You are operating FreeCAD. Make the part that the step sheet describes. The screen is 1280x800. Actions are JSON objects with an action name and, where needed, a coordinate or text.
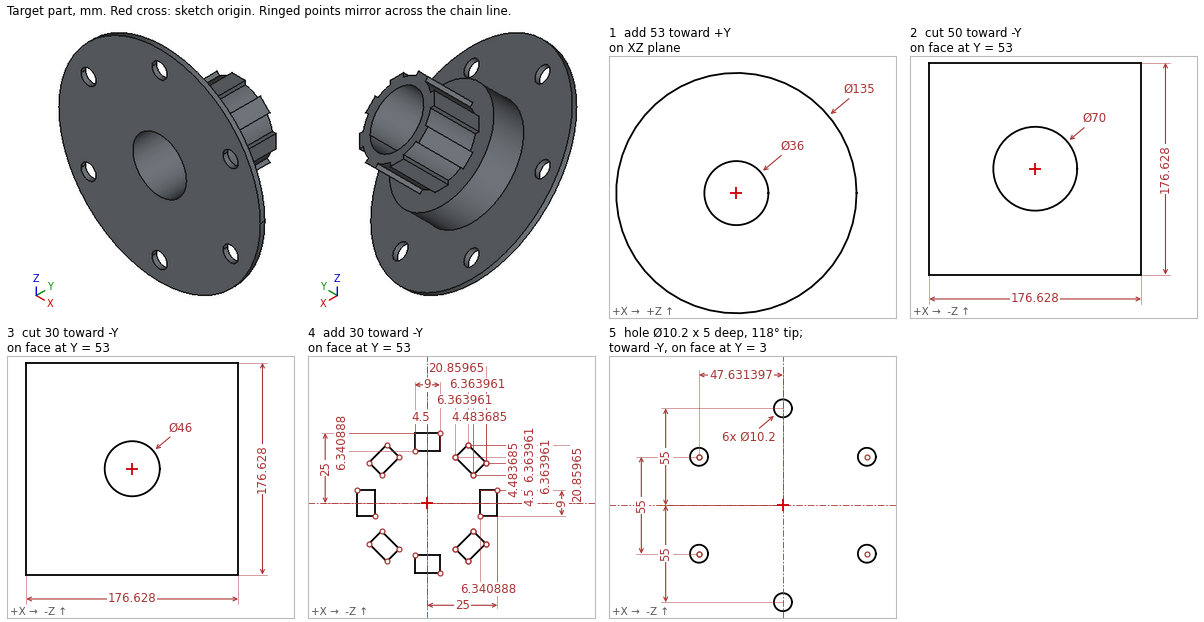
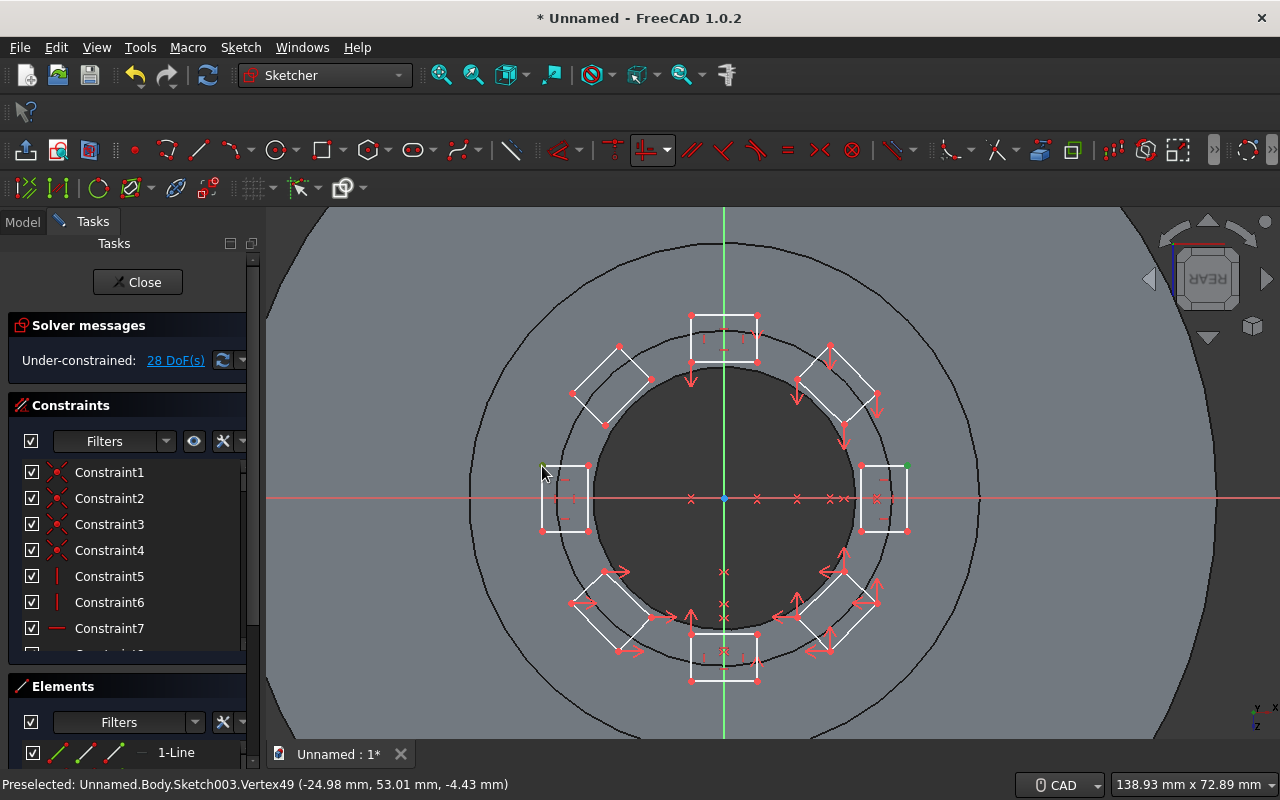
{"action": "left_click", "coordinate": [724, 541]}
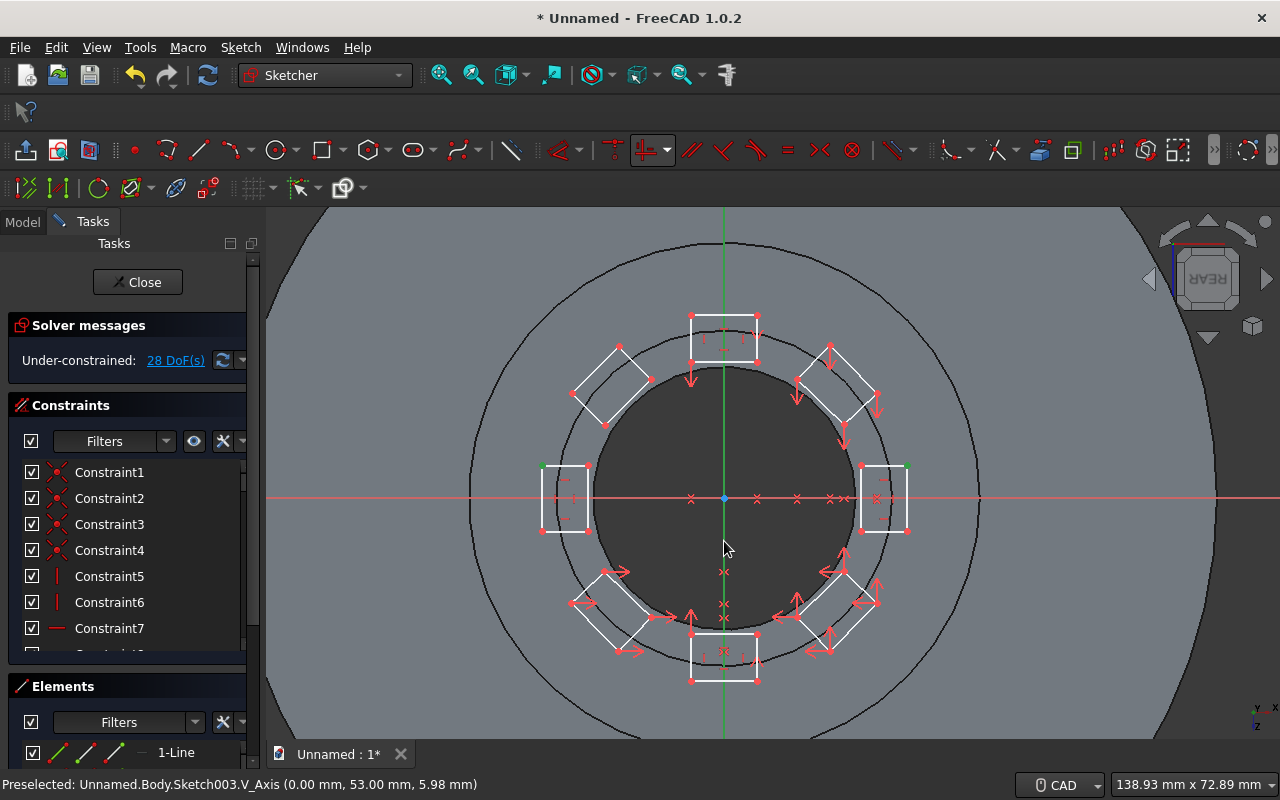
{"action": "left_click", "coordinate": [820, 150]}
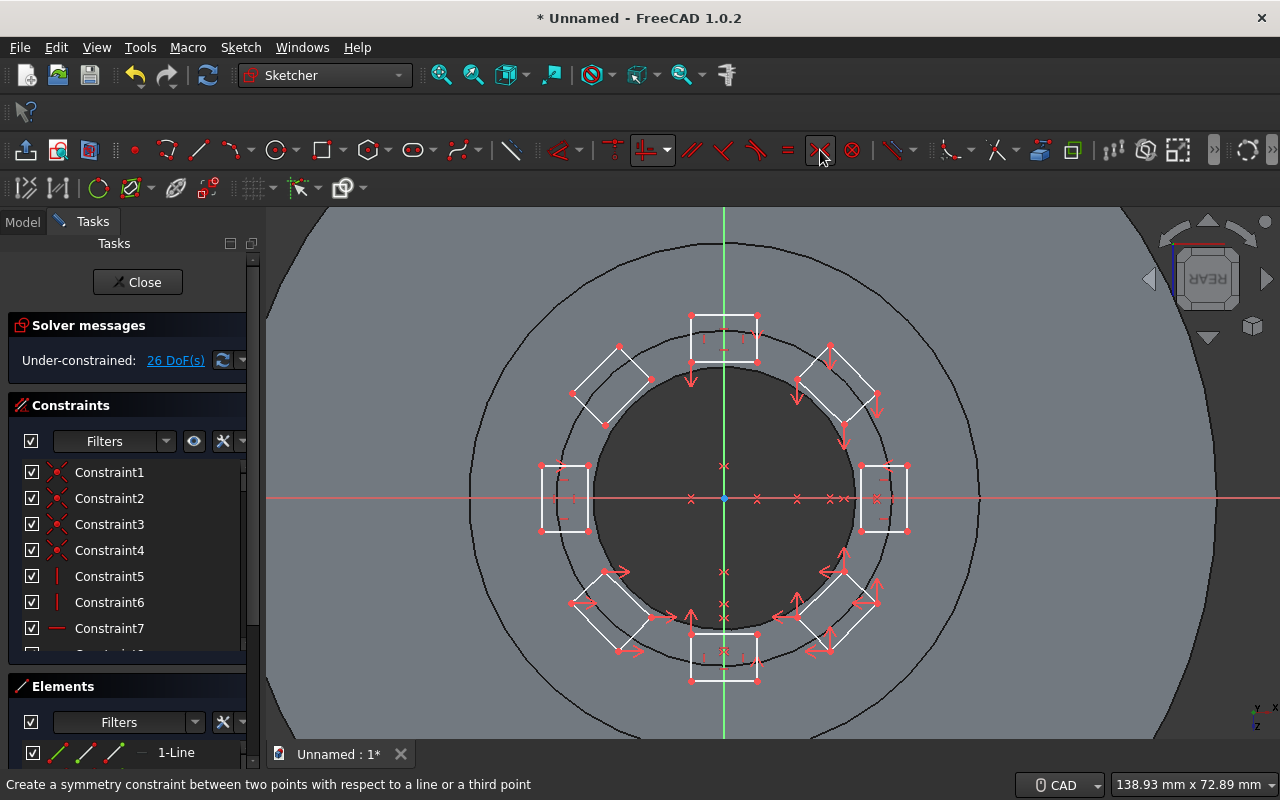
{"action": "left_click", "coordinate": [861, 532]}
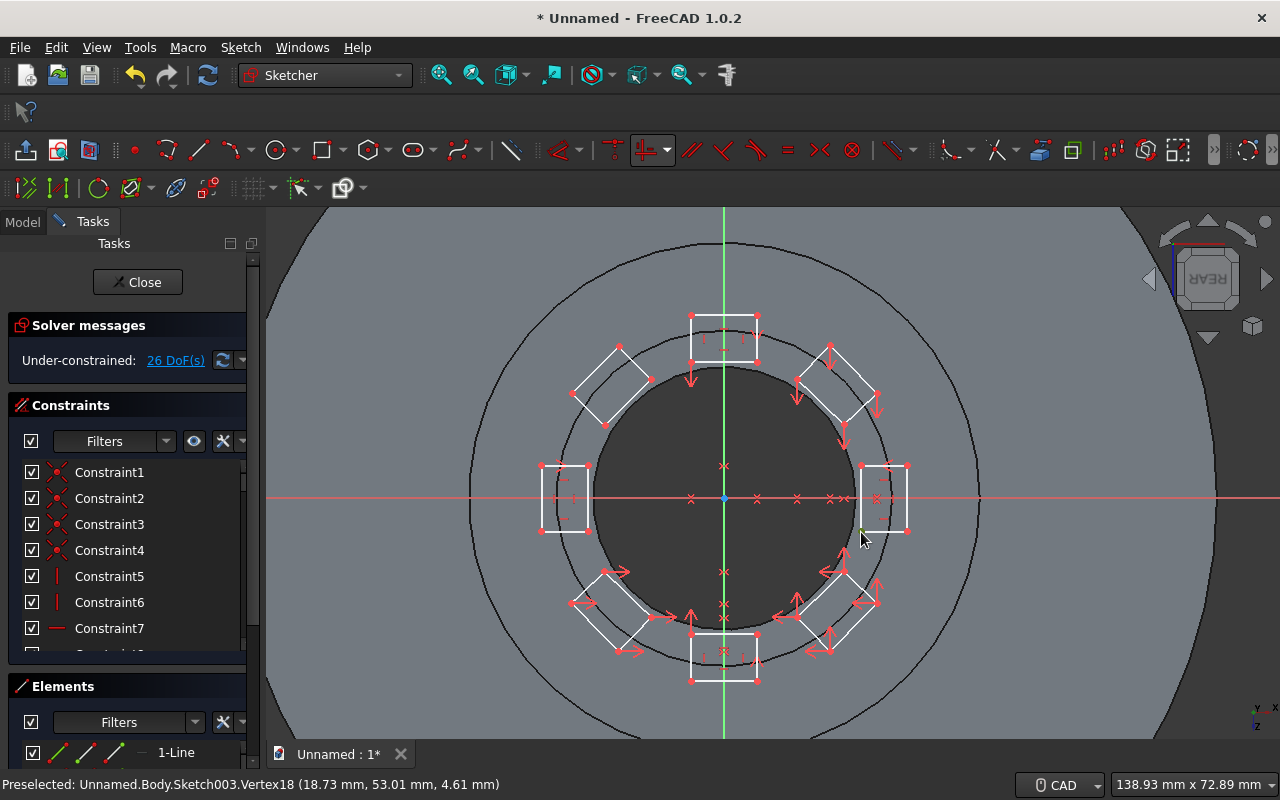
{"action": "left_click", "coordinate": [588, 532]}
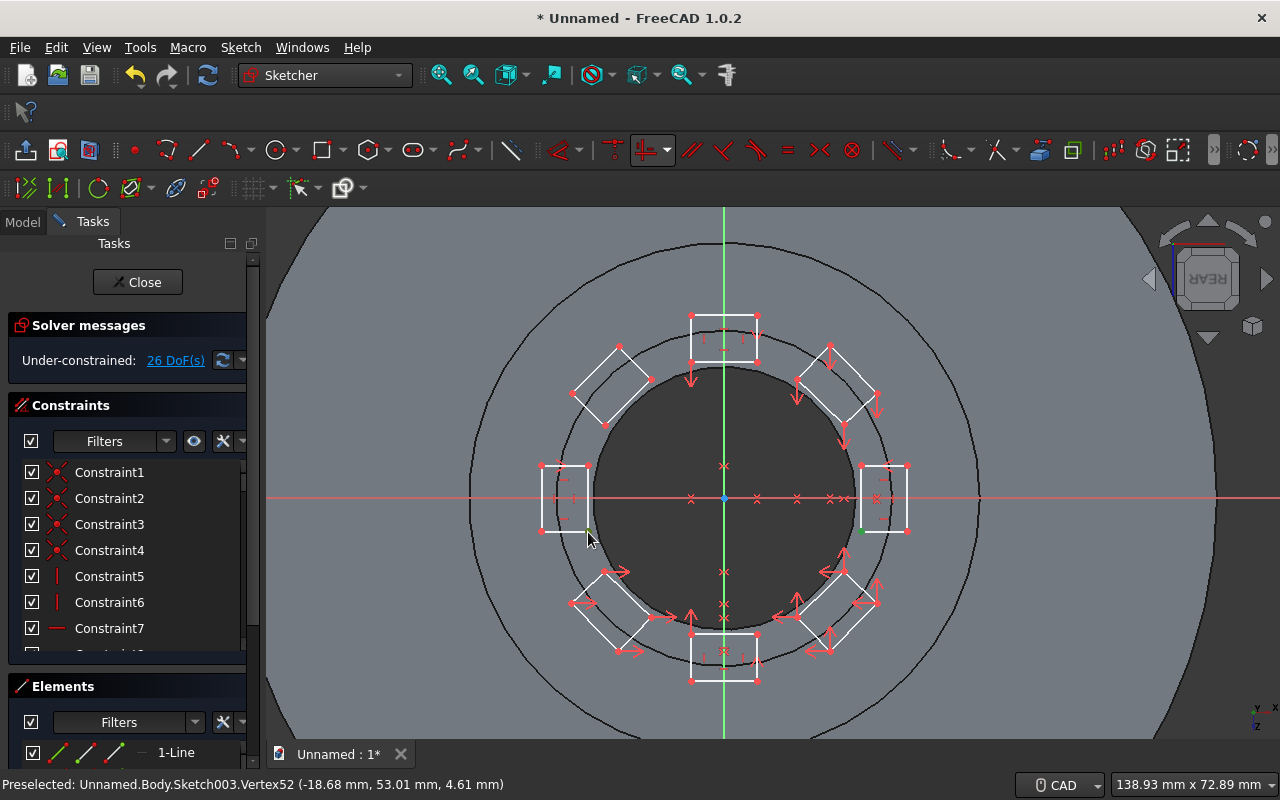
{"action": "left_click", "coordinate": [724, 541]}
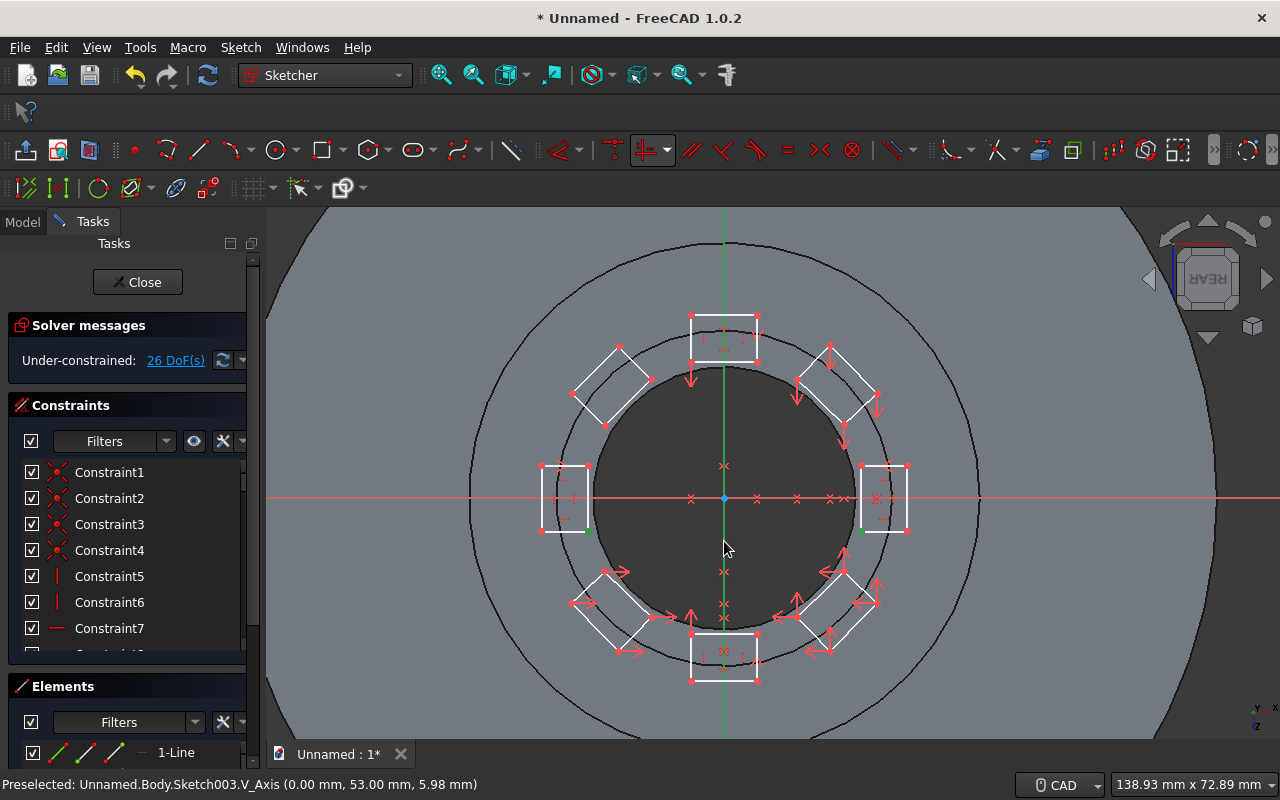
{"action": "left_click", "coordinate": [820, 150]}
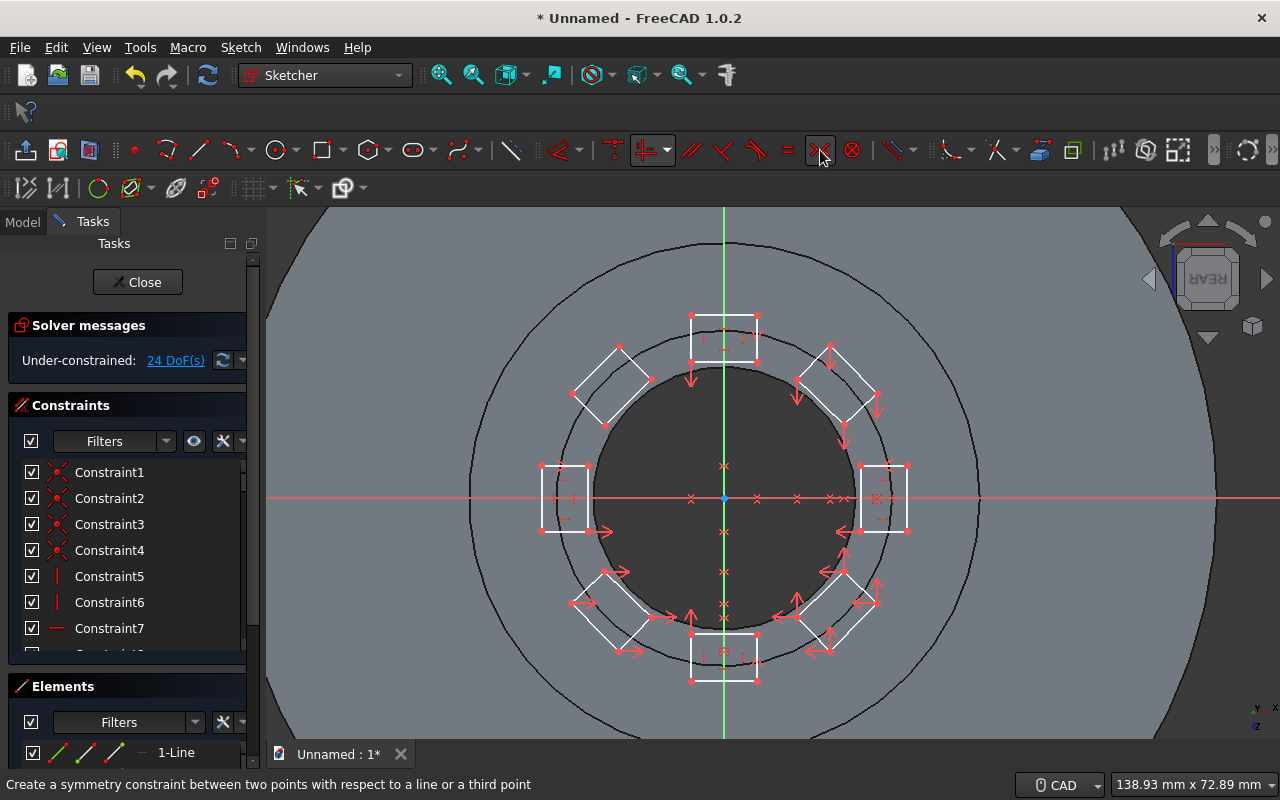
{"action": "left_click", "coordinate": [844, 425]}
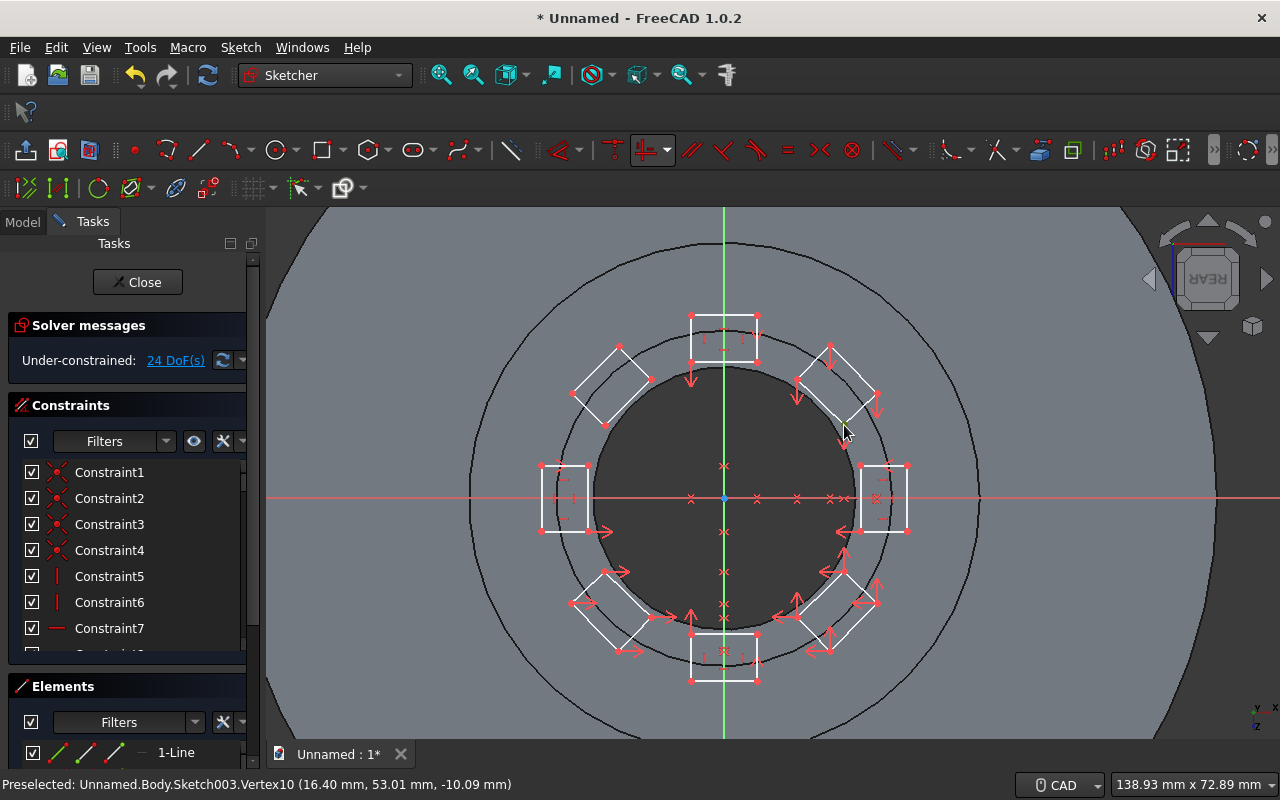
{"action": "left_click", "coordinate": [605, 426]}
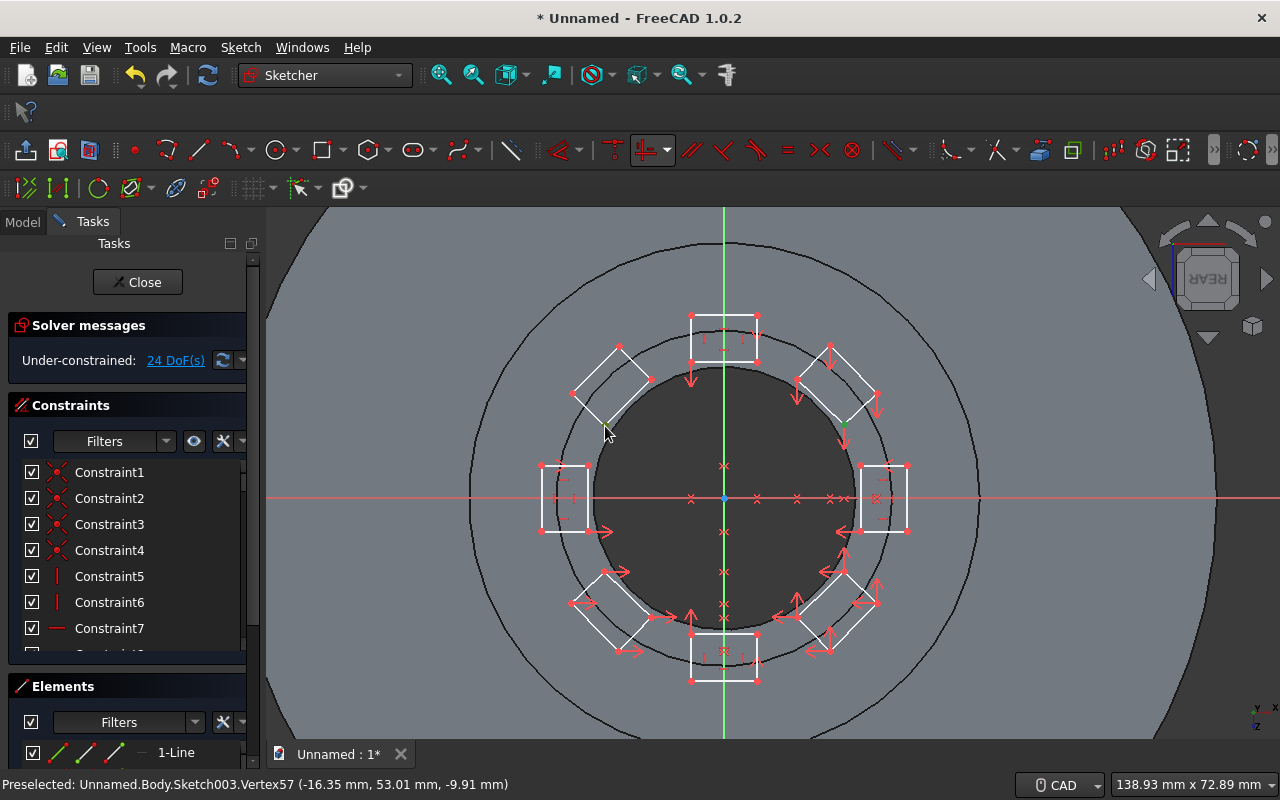
{"action": "left_click", "coordinate": [724, 541]}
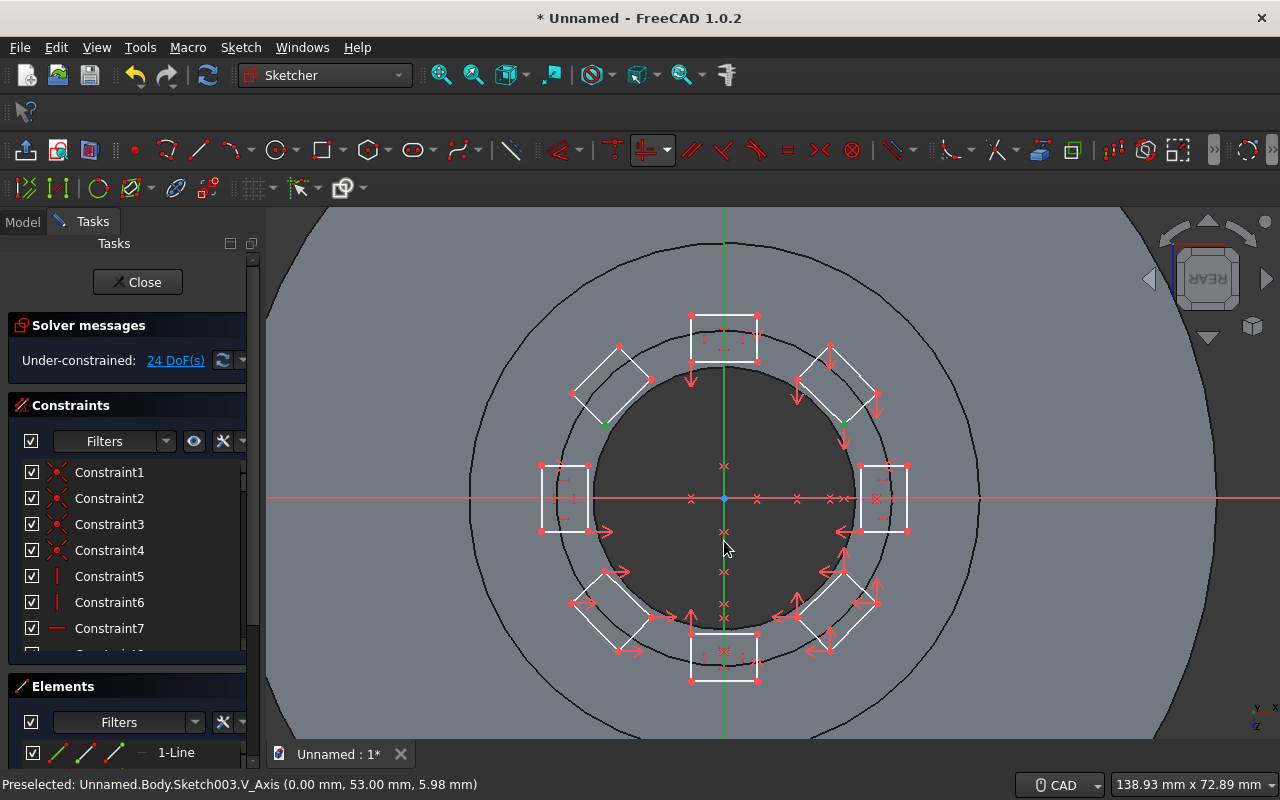
{"action": "left_click", "coordinate": [820, 150]}